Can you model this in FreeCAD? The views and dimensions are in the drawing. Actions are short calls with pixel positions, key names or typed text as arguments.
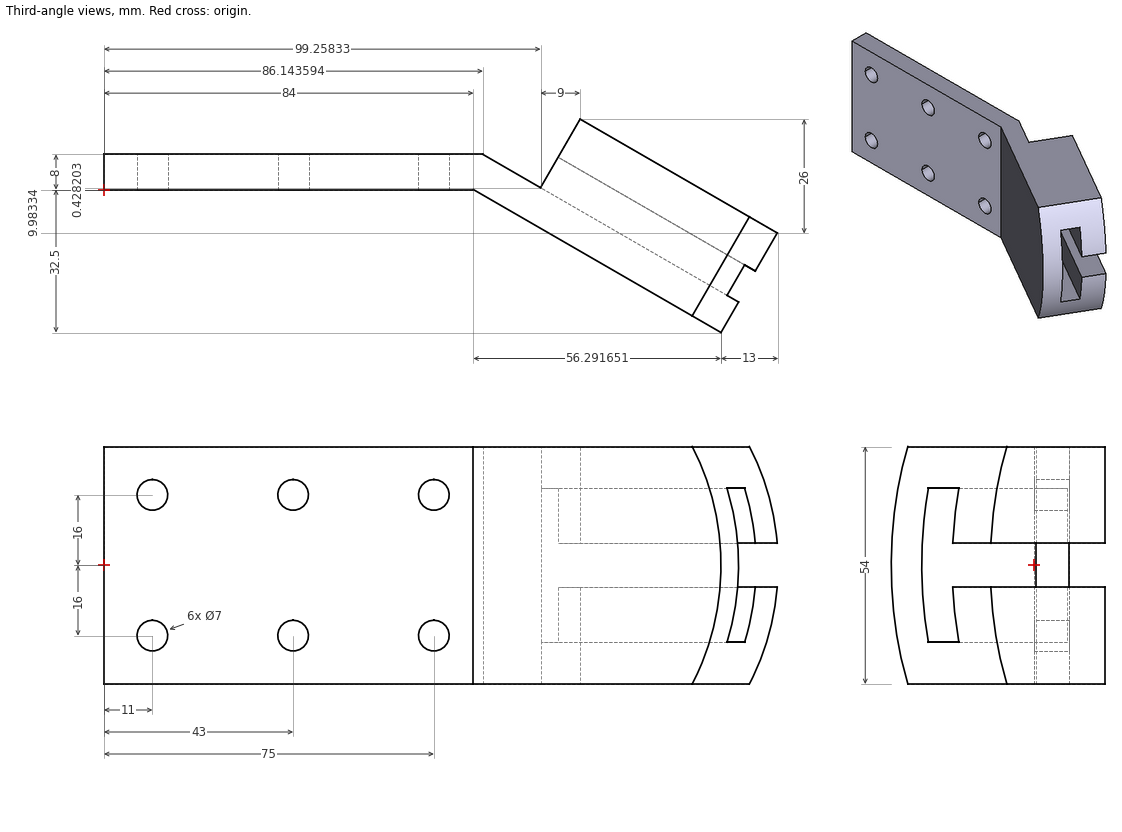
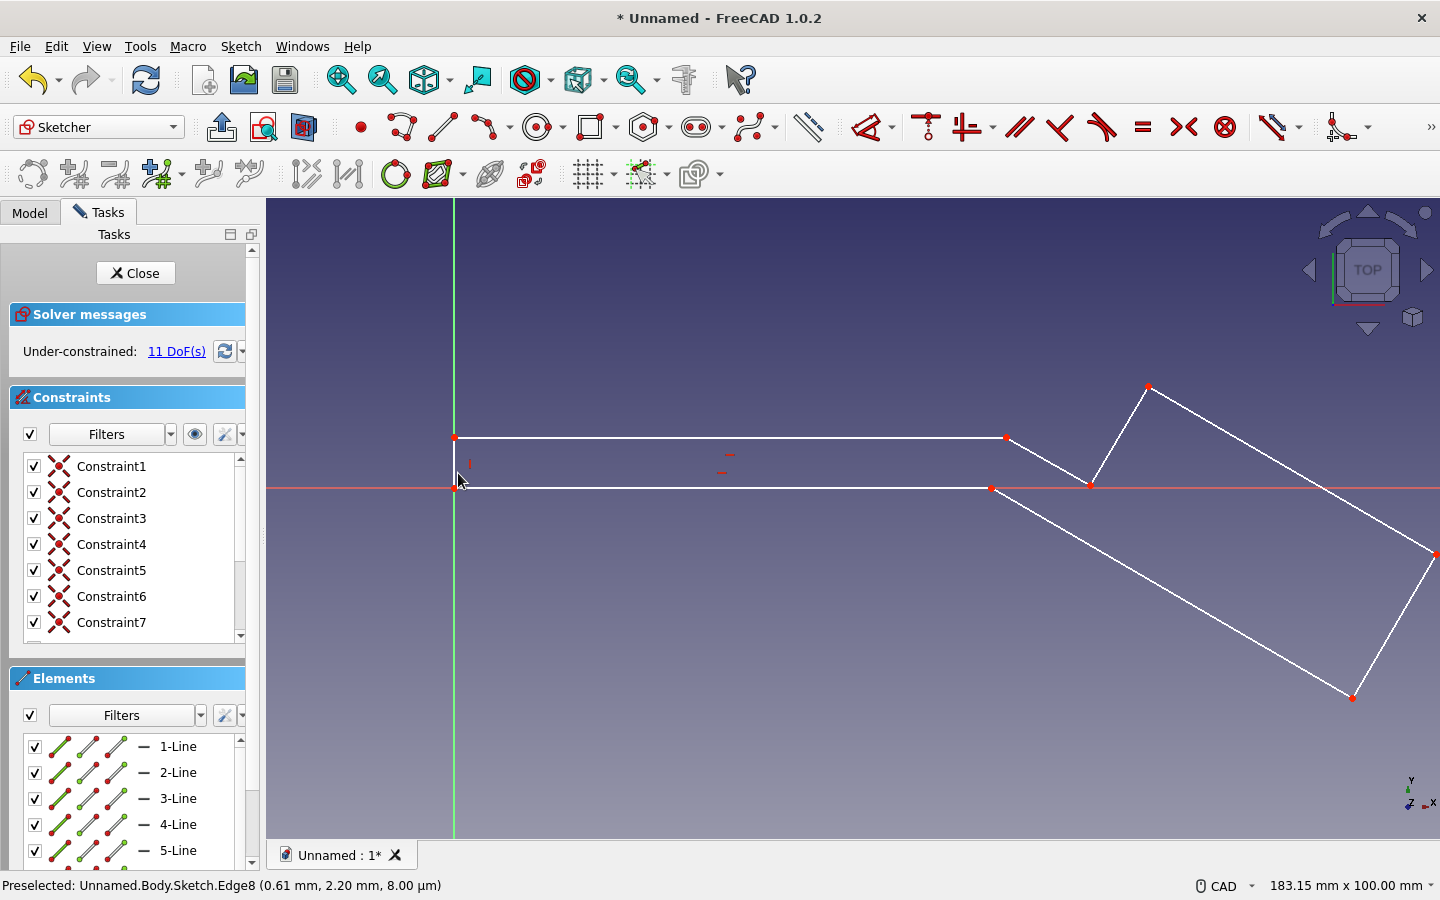
key(d)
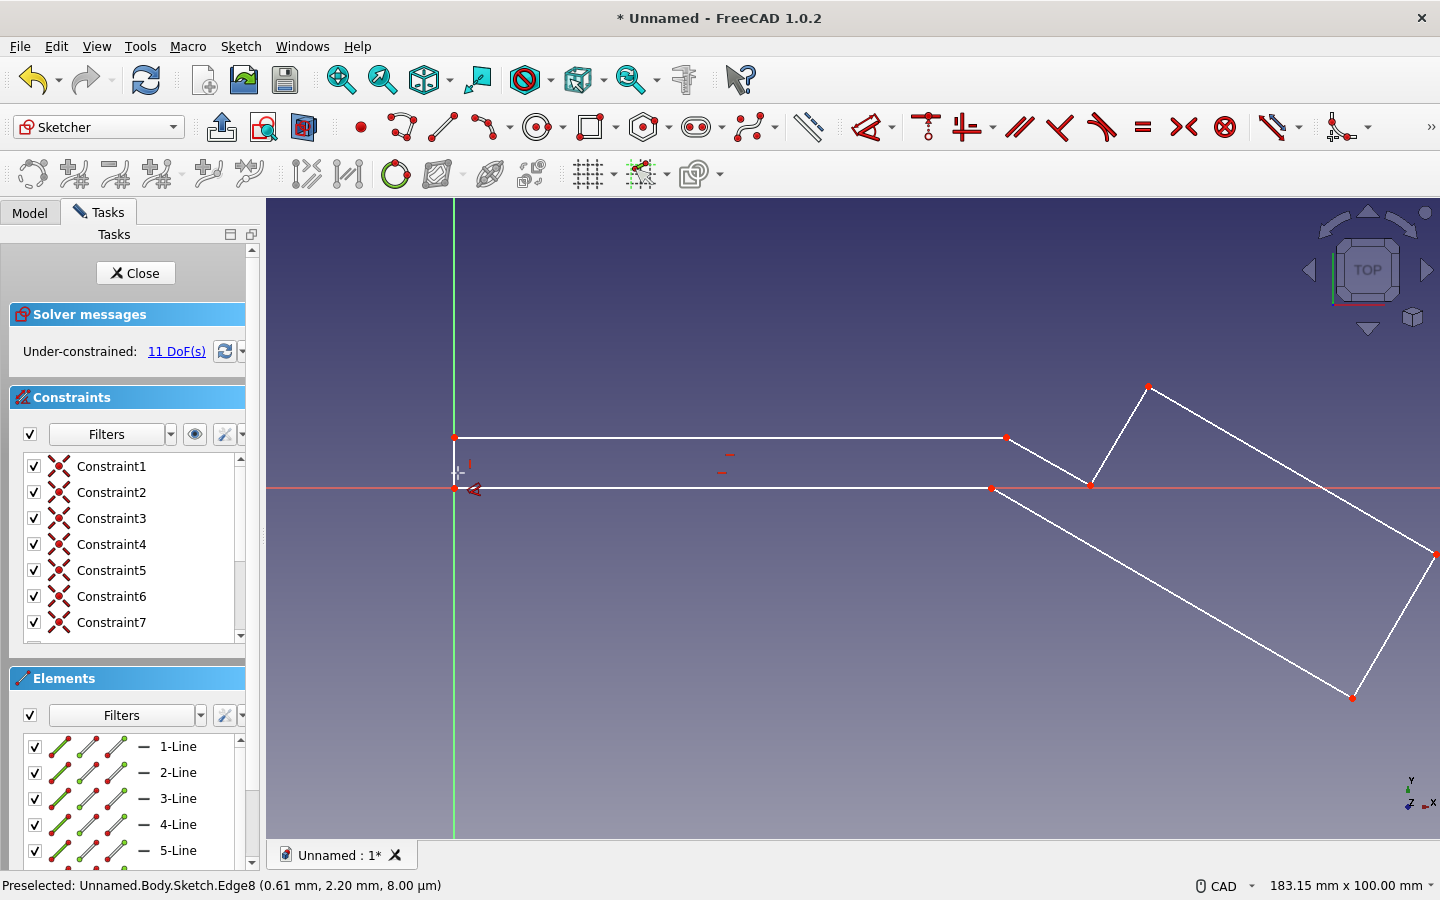
click(454, 453)
click(420, 463)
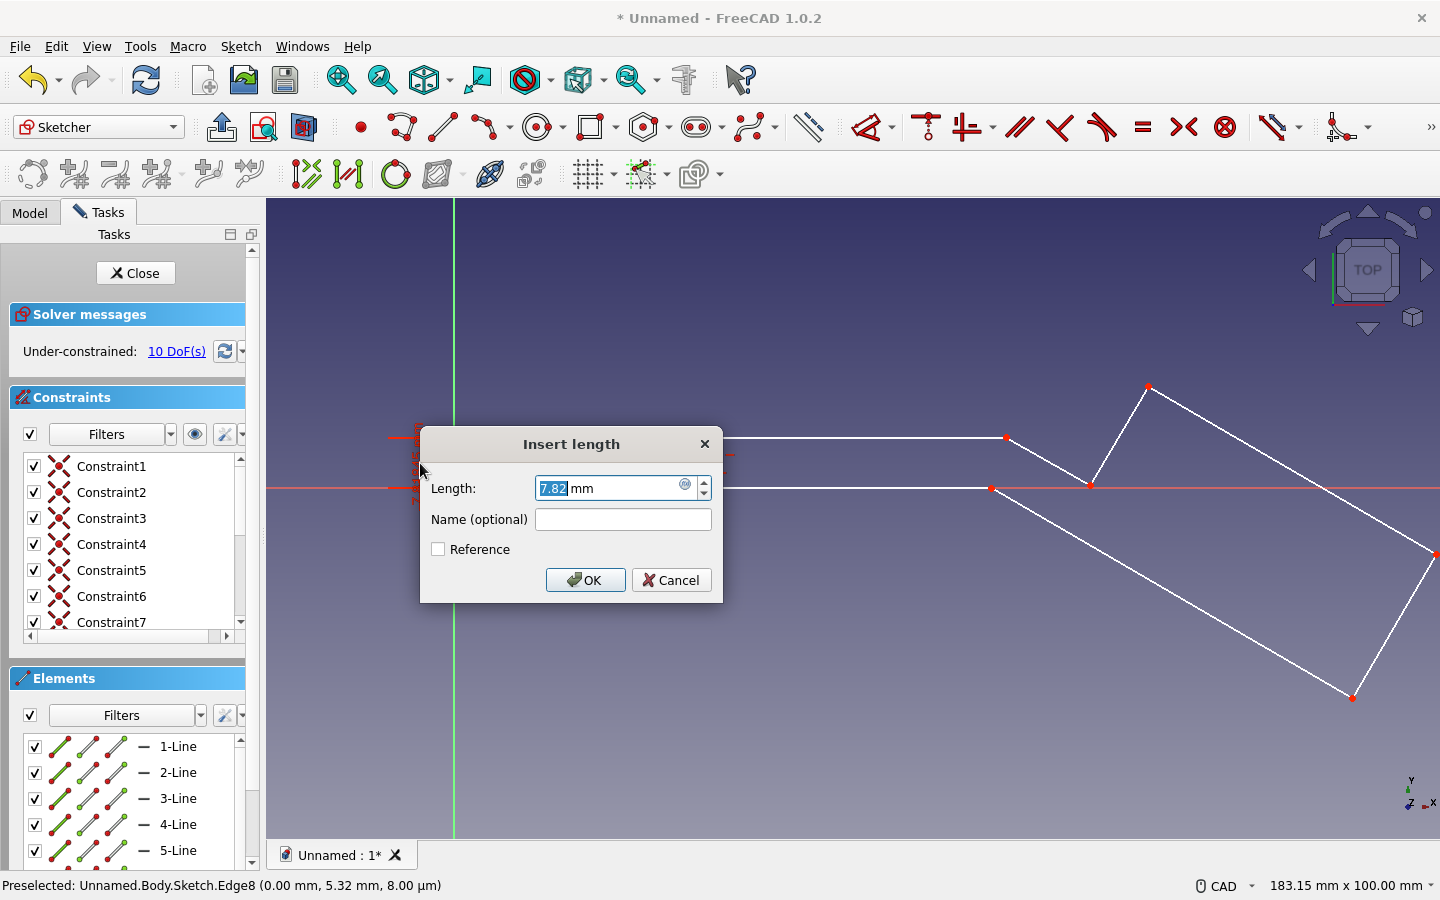
text(8)
key(Return)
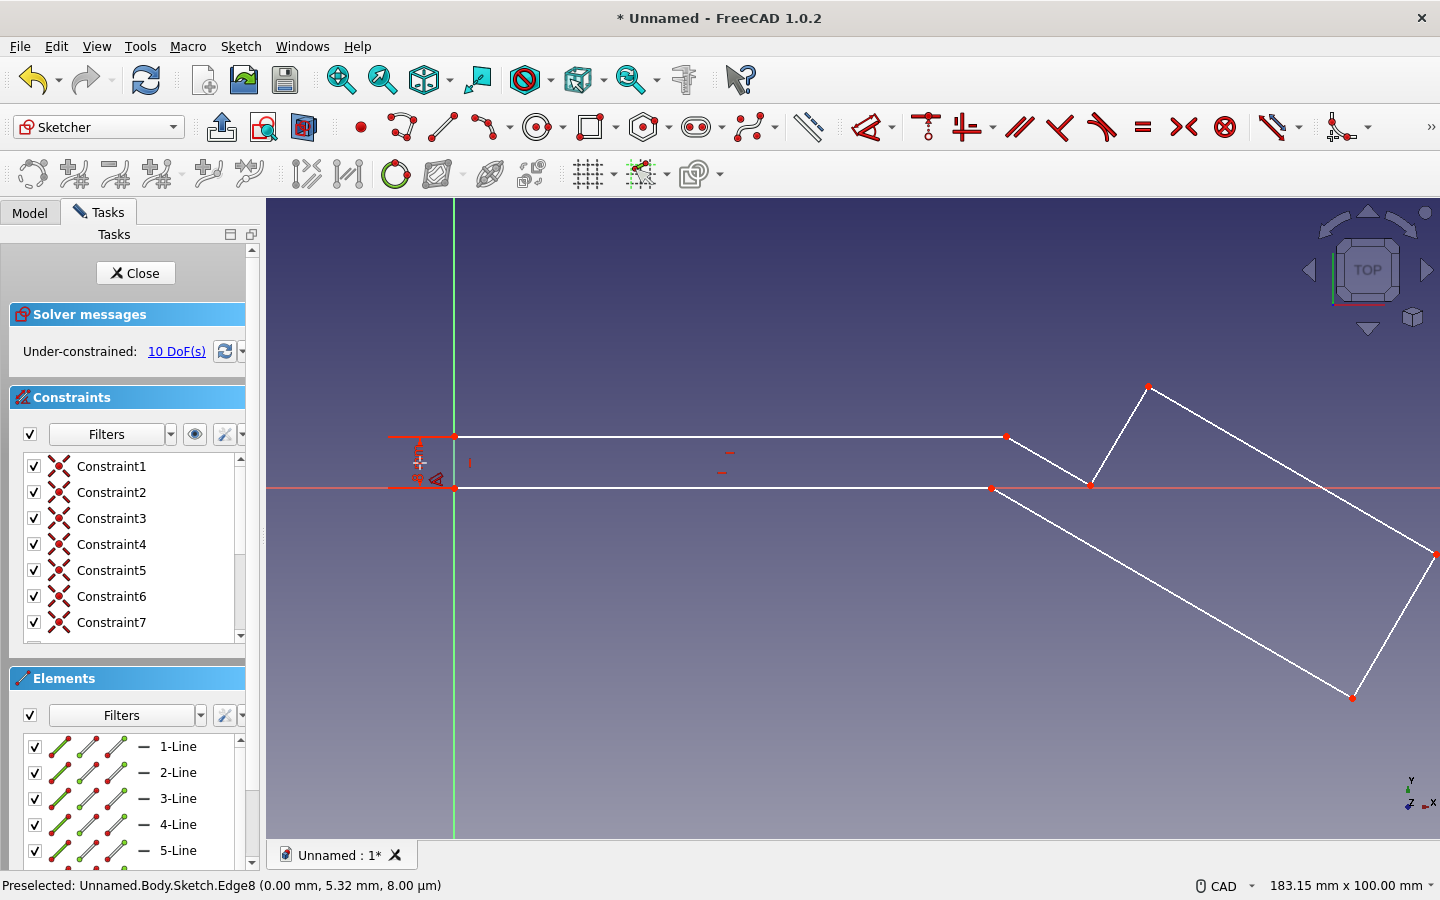
click(615, 488)
click(723, 454)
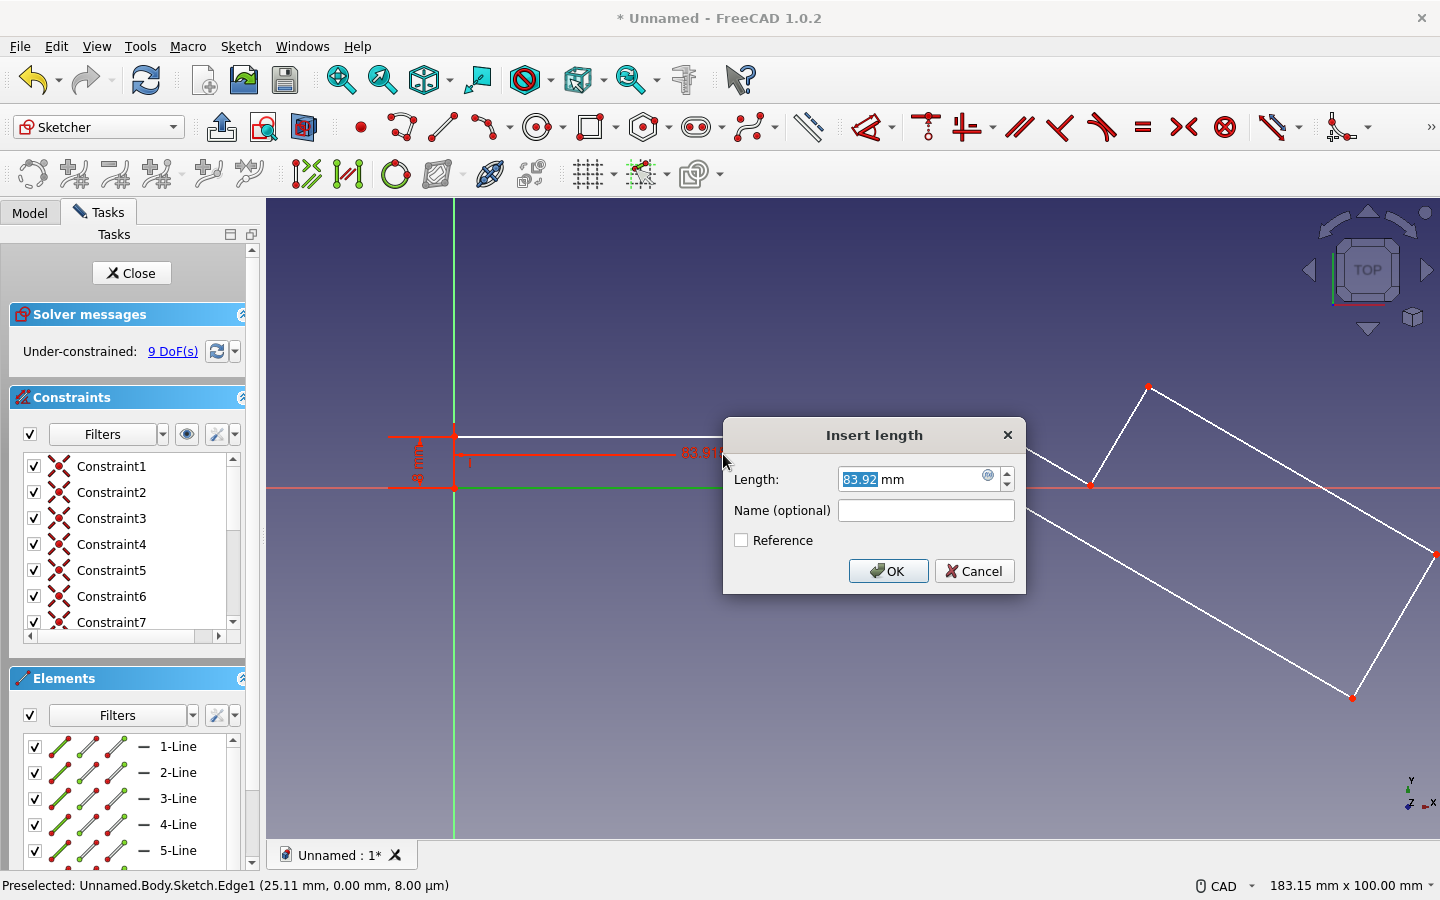
text(84)
key(Return)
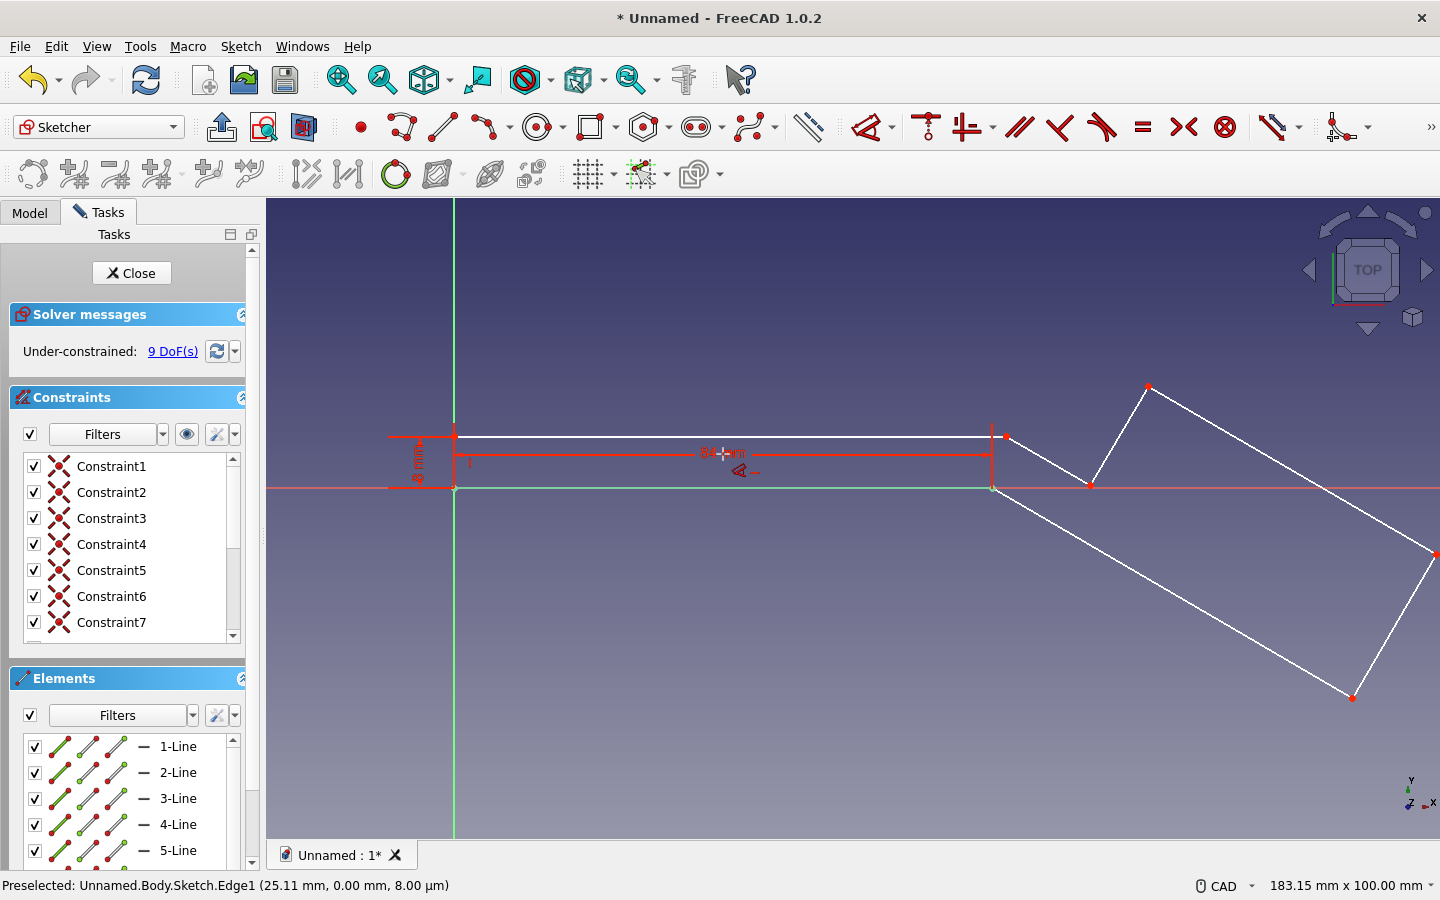
click(1131, 416)
click(1119, 353)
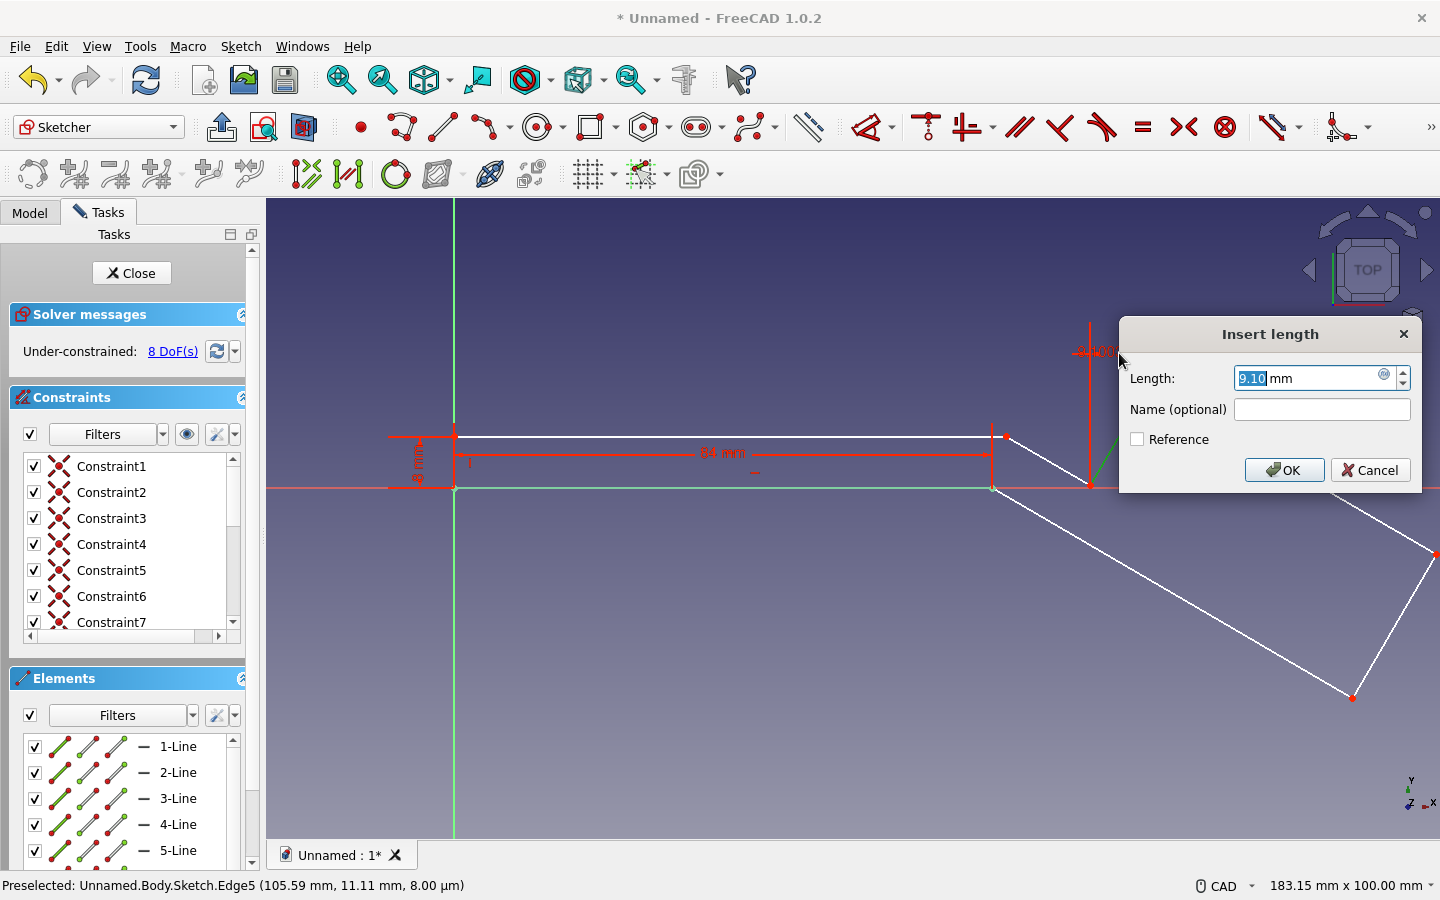
text(9)
key(Return)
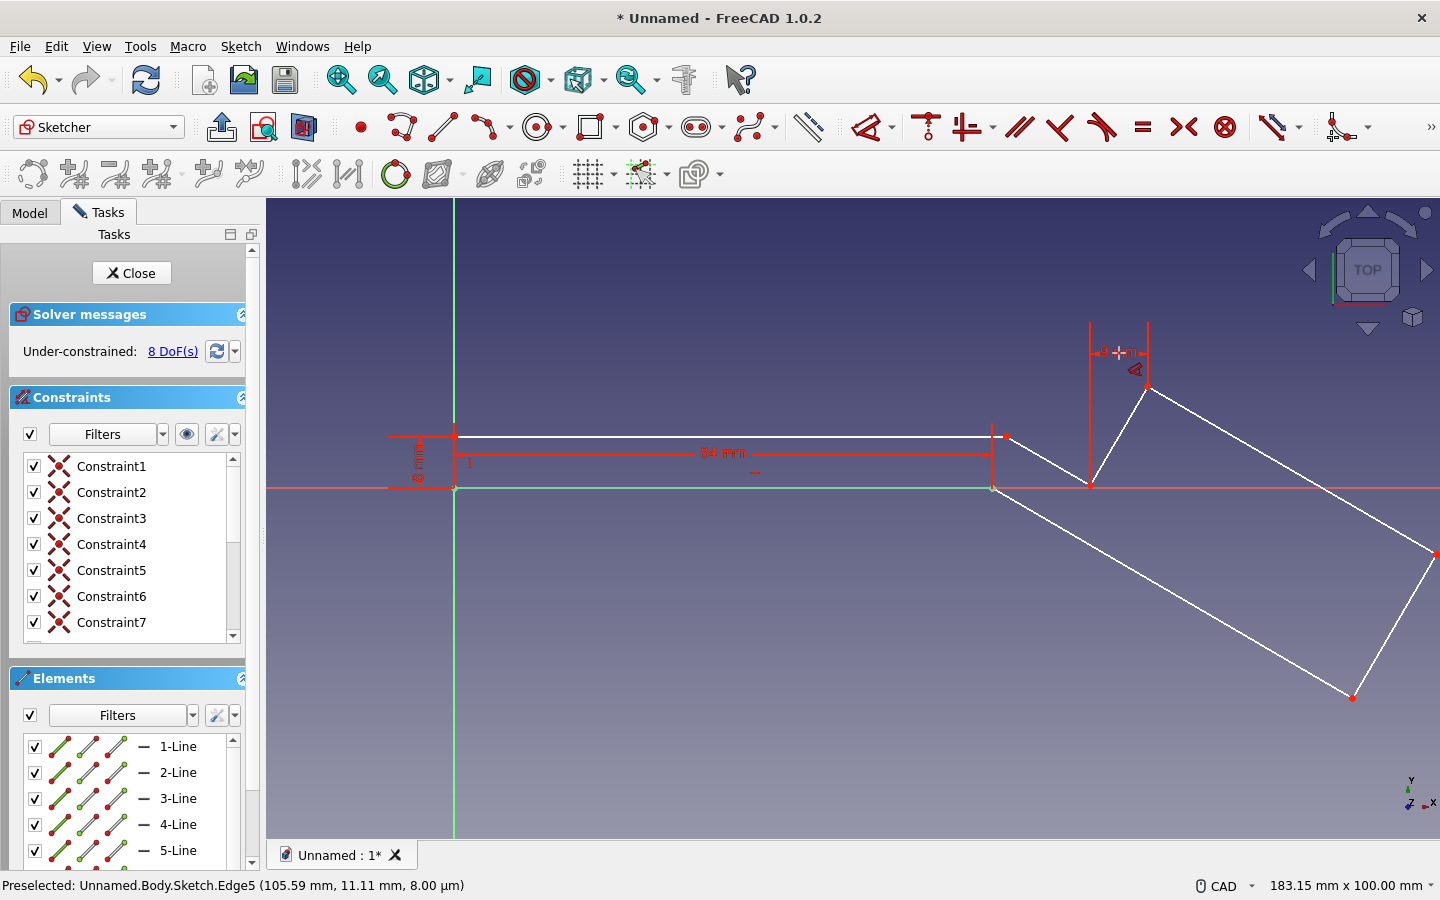
scroll(458, 473, down, 2)